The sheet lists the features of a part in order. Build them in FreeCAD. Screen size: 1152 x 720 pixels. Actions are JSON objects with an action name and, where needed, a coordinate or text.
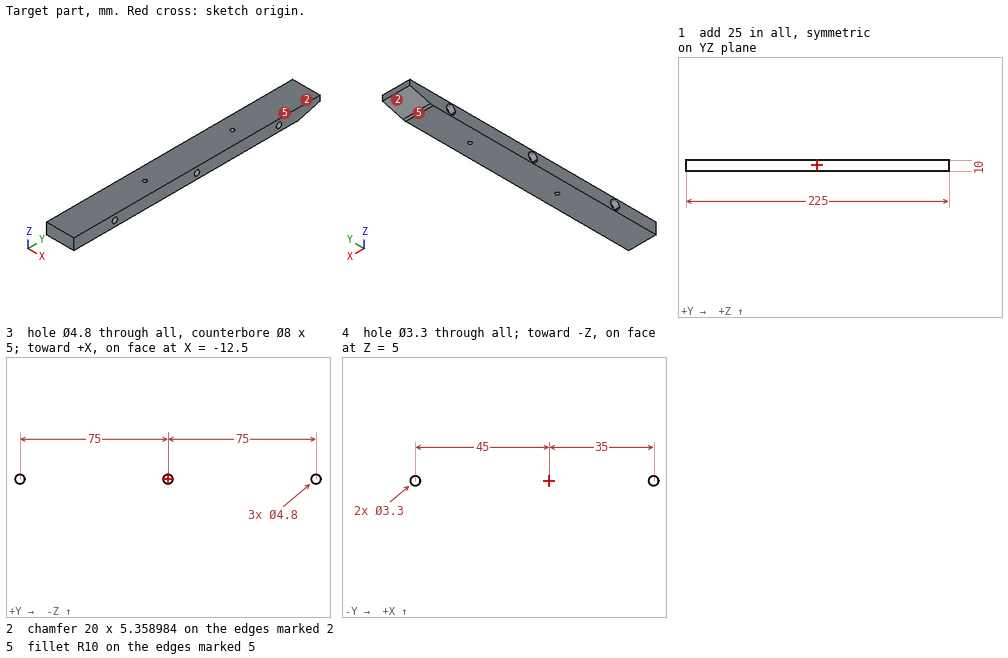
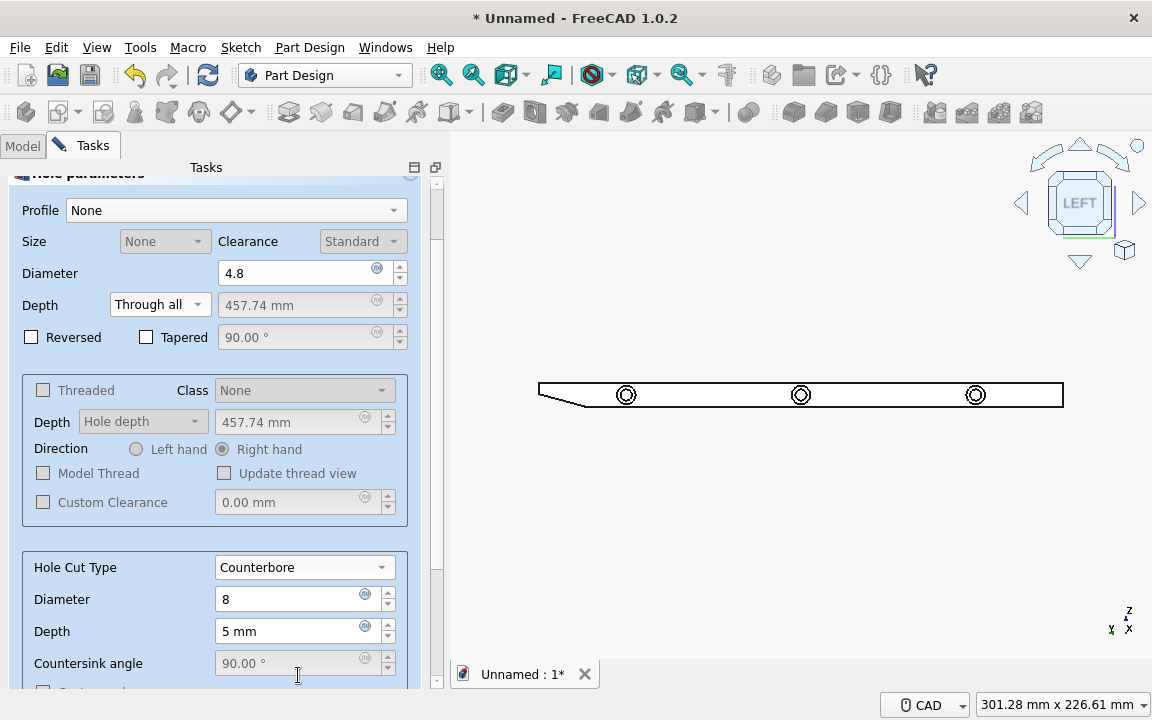
{"action": "scroll", "coordinate": [437, 432], "scroll_direction": "up", "scroll_amount": 3}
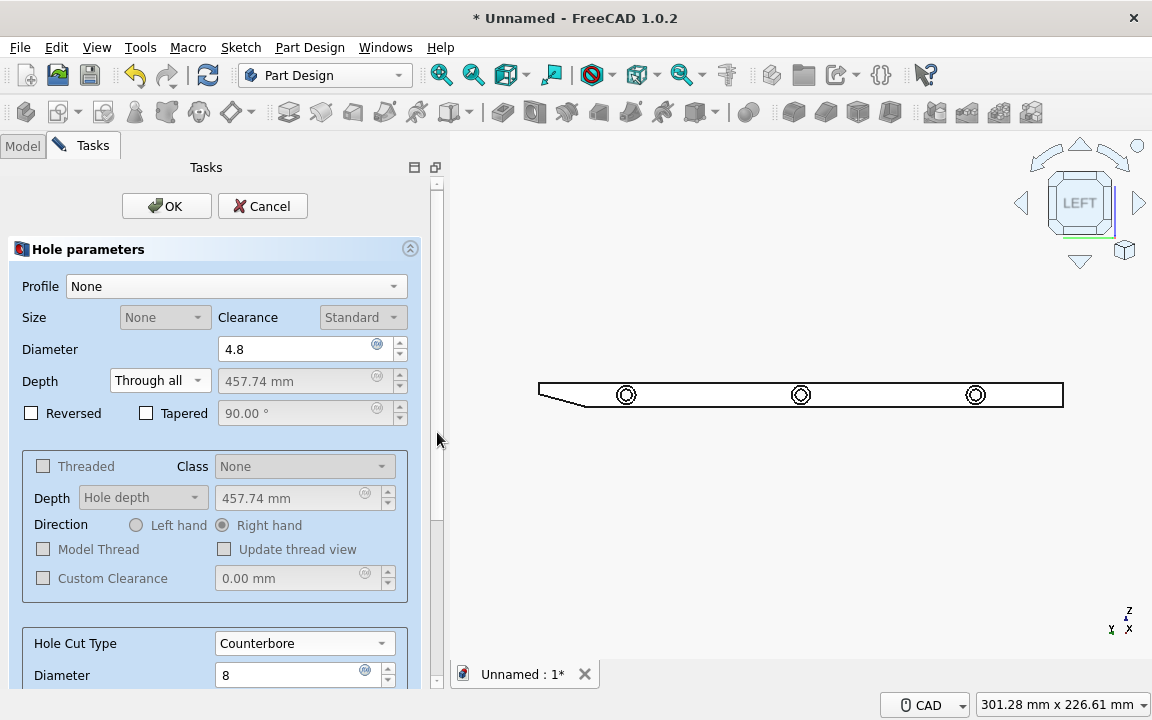
{"action": "left_click", "coordinate": [167, 206]}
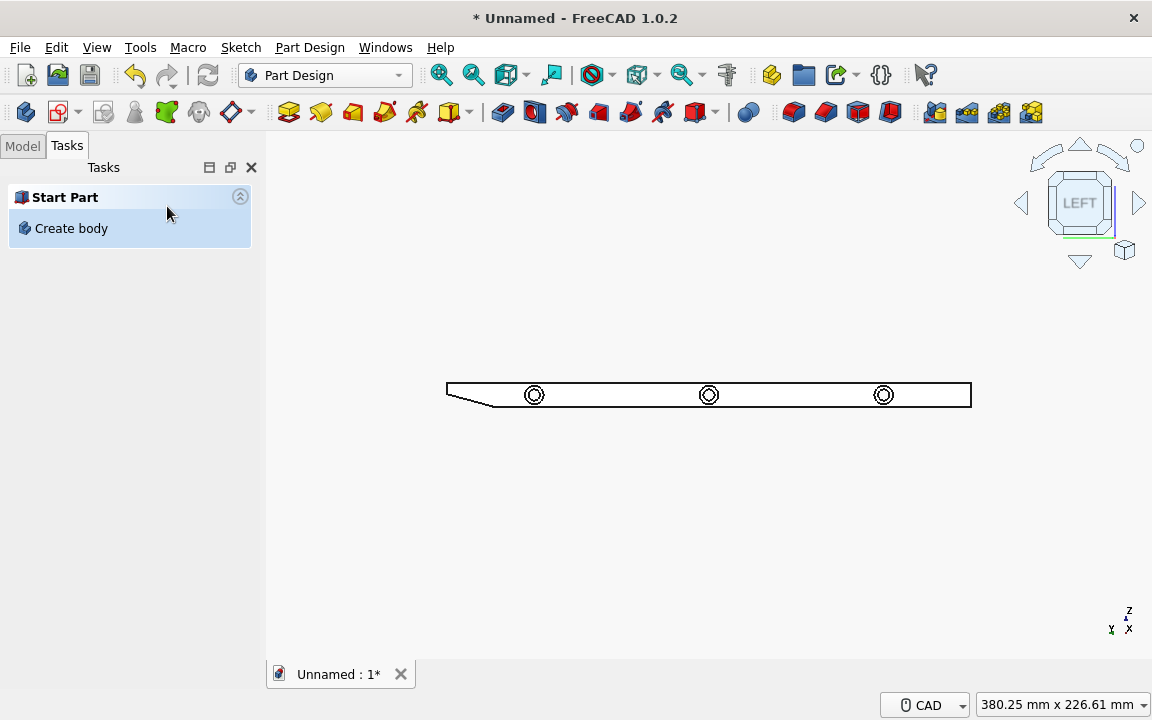
{"action": "key", "text": "0"}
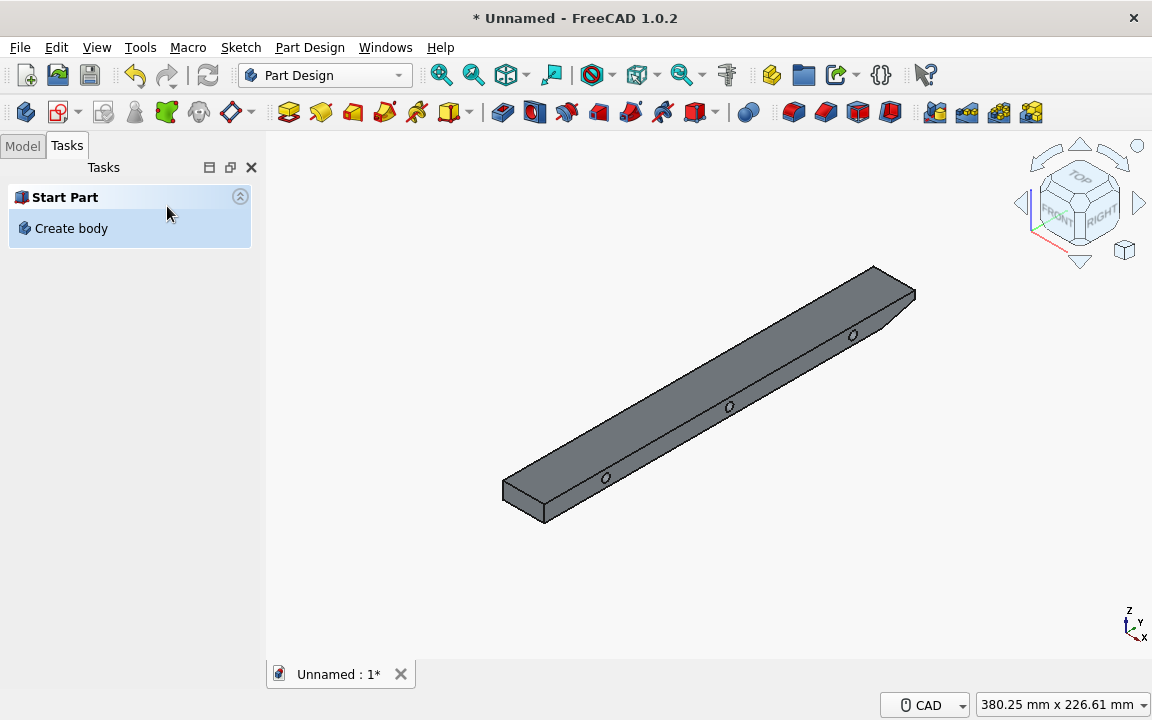
{"action": "left_click", "coordinate": [868, 293]}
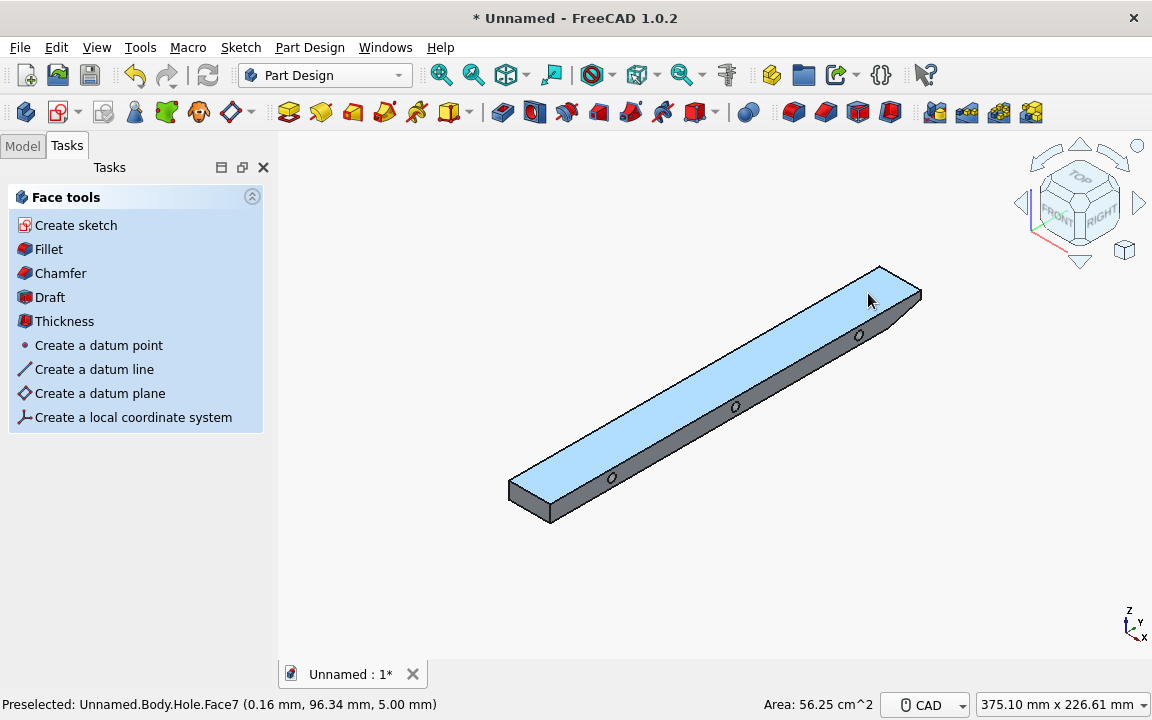
{"action": "left_click", "coordinate": [58, 112]}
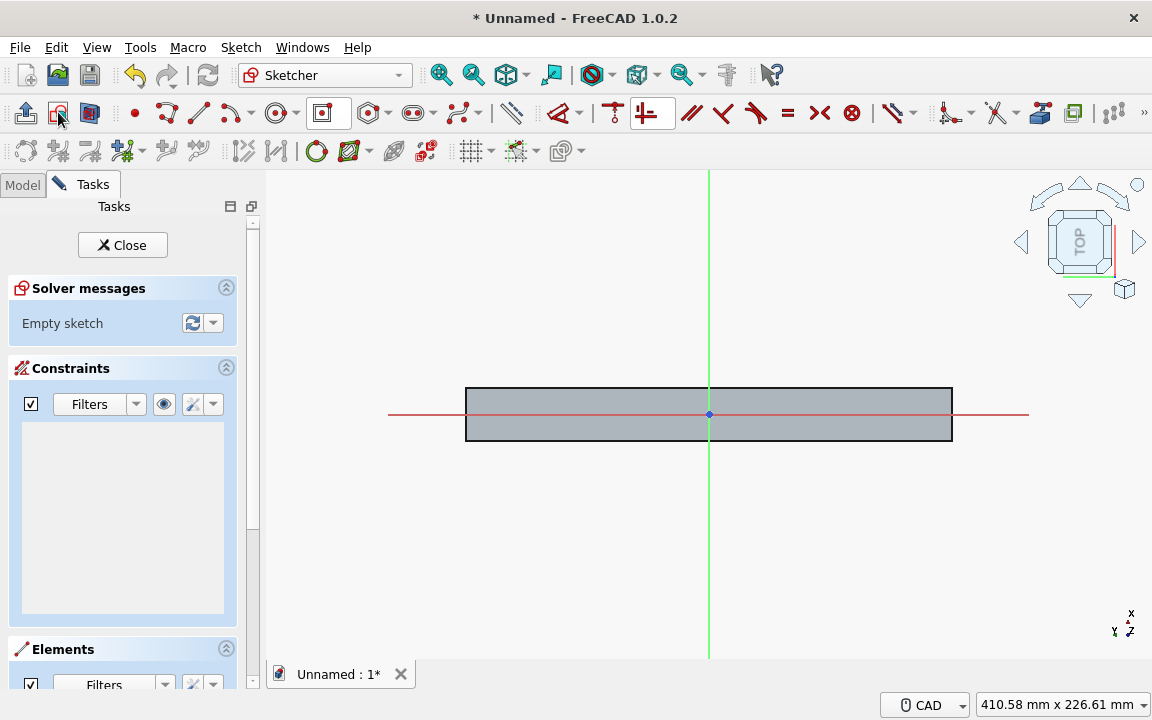
{"action": "scroll", "coordinate": [732, 415], "scroll_direction": "up", "scroll_amount": 5}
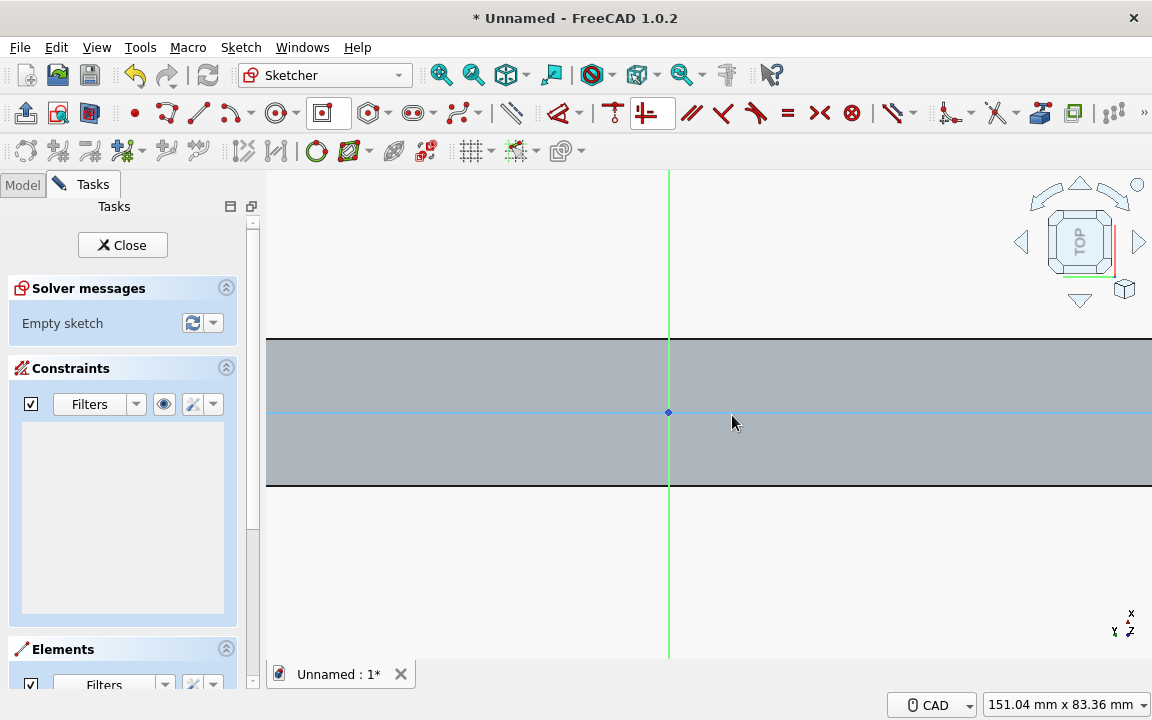
{"action": "left_click", "coordinate": [276, 114]}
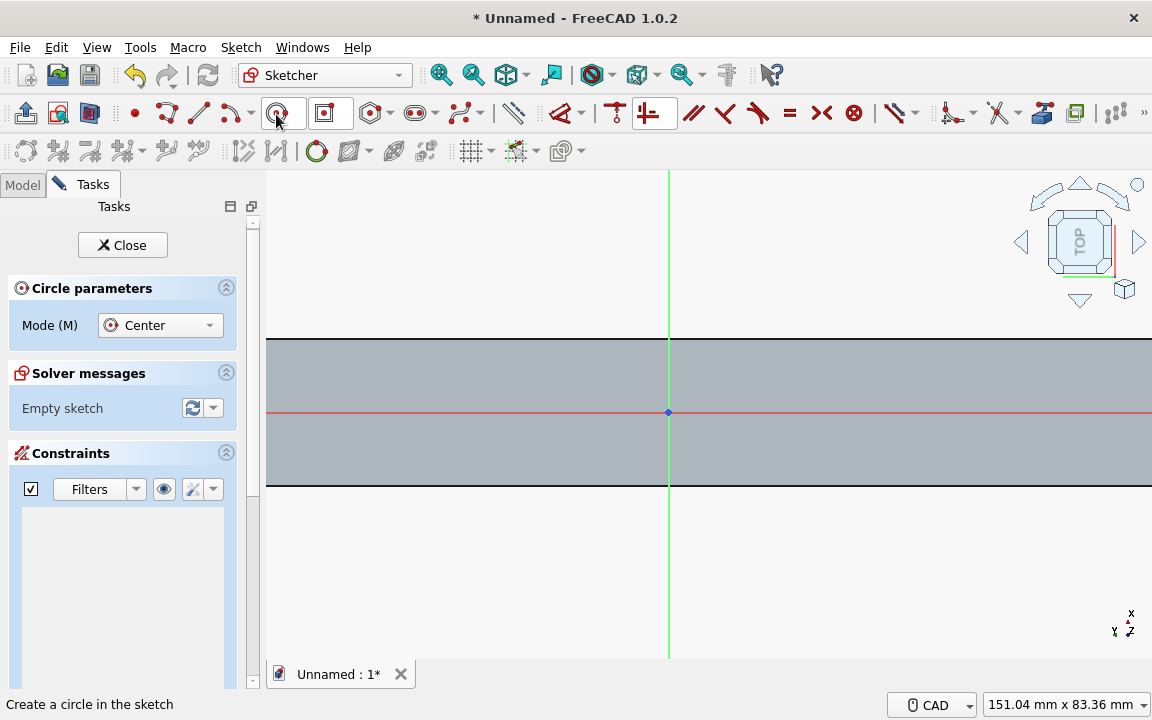
{"action": "scroll", "coordinate": [405, 413], "scroll_direction": "up", "scroll_amount": 5}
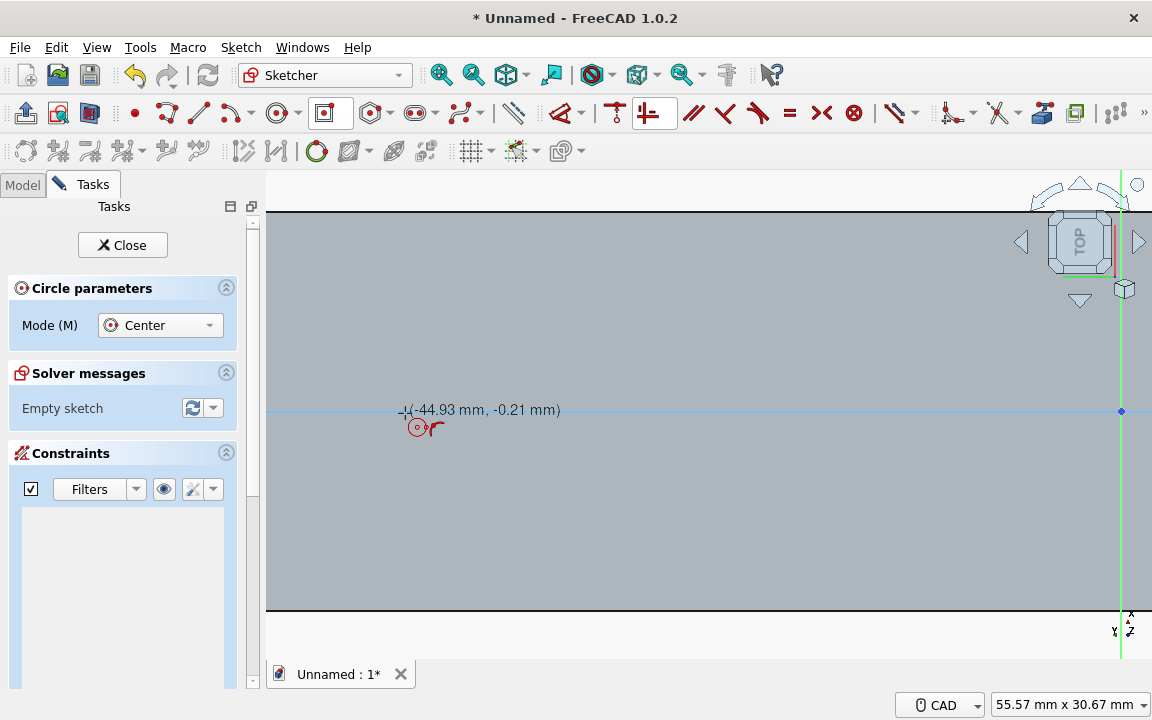
{"action": "left_click", "coordinate": [404, 412]}
{"action": "left_click", "coordinate": [422, 393]}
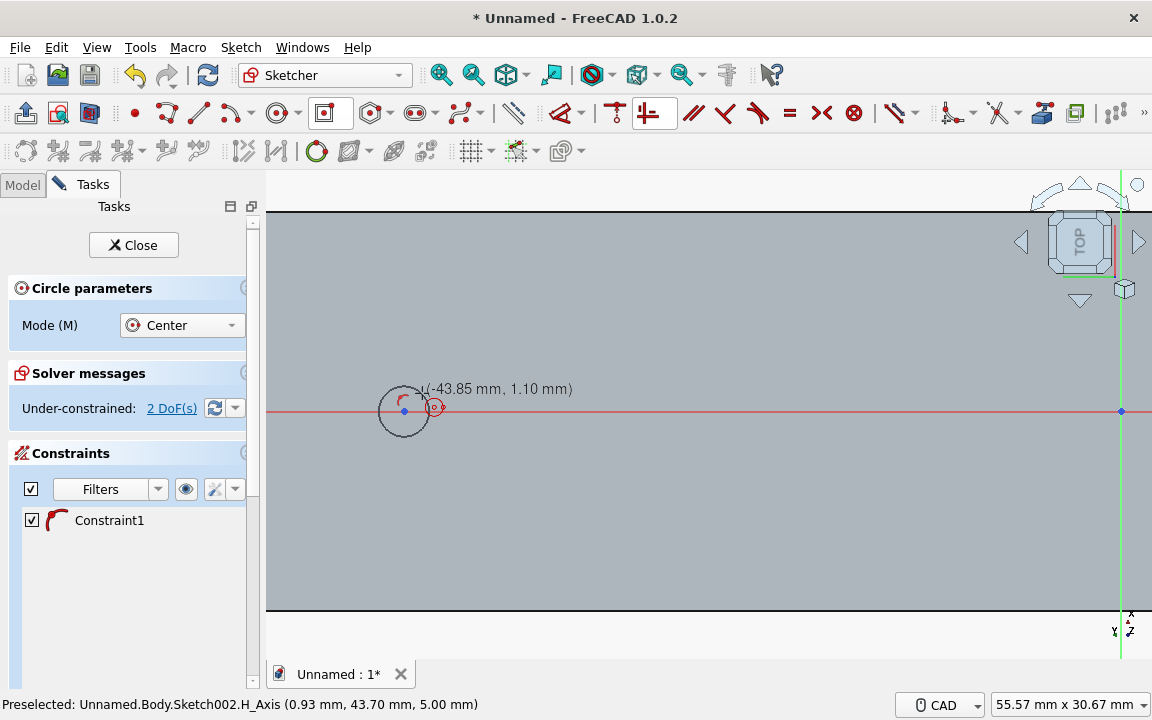
{"action": "scroll", "coordinate": [407, 416], "scroll_direction": "down", "scroll_amount": 5}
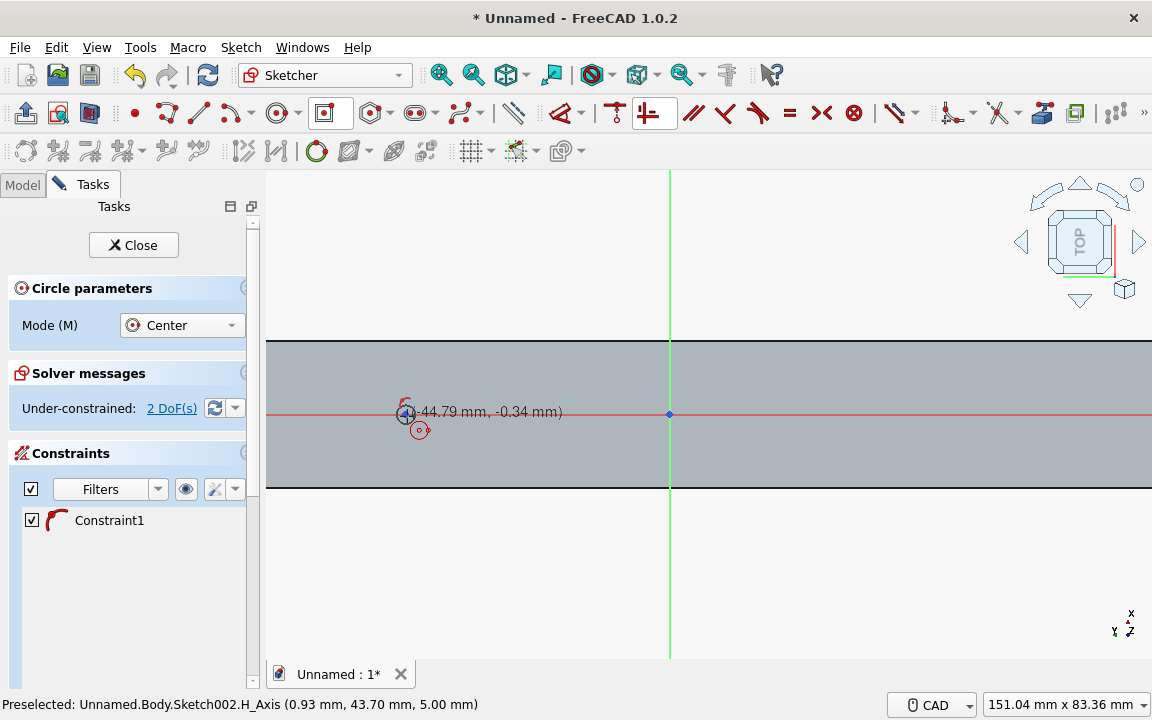
{"action": "scroll", "coordinate": [875, 415], "scroll_direction": "up", "scroll_amount": 5}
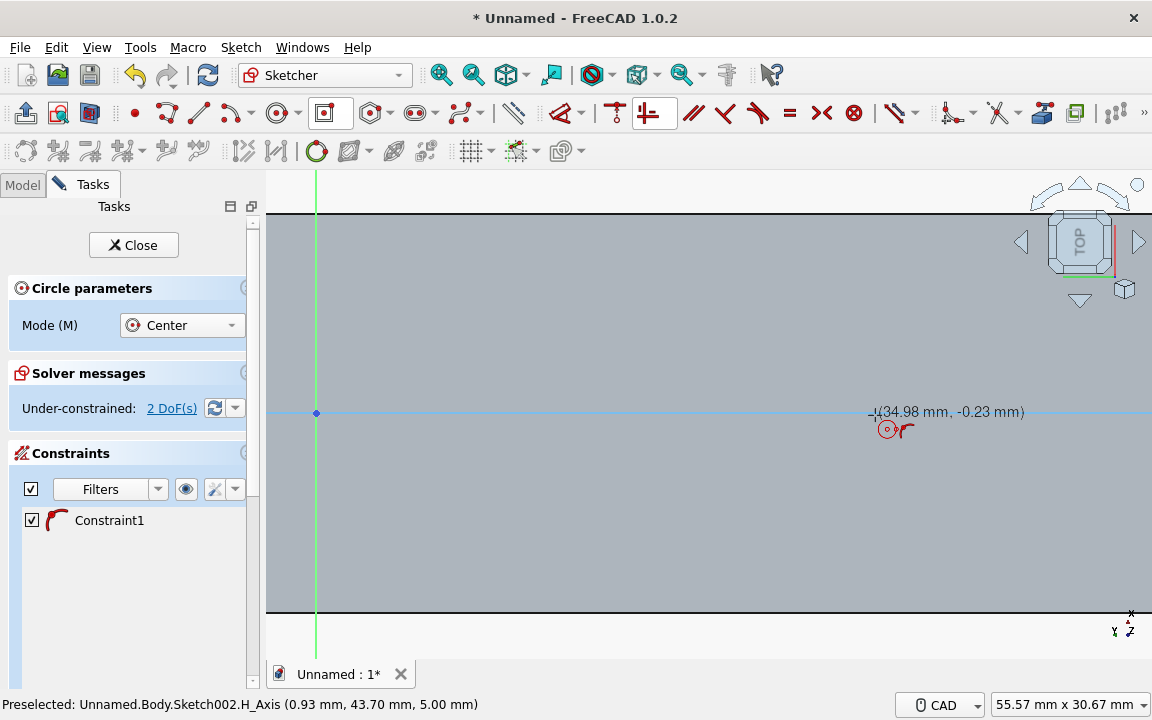
{"action": "left_click", "coordinate": [874, 413]}
{"action": "left_click", "coordinate": [893, 395]}
{"action": "key", "text": "Escape"}